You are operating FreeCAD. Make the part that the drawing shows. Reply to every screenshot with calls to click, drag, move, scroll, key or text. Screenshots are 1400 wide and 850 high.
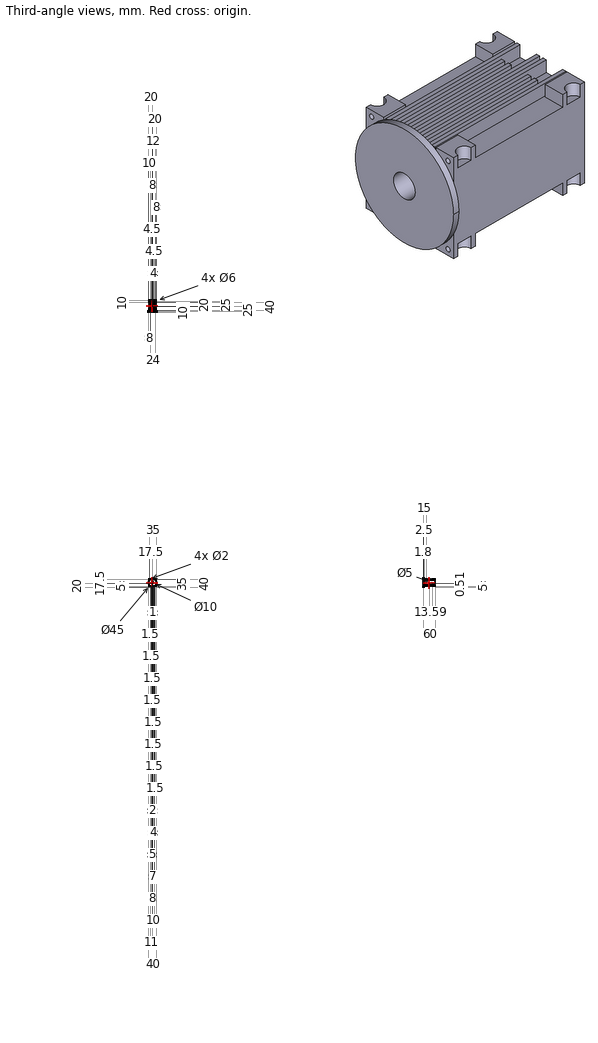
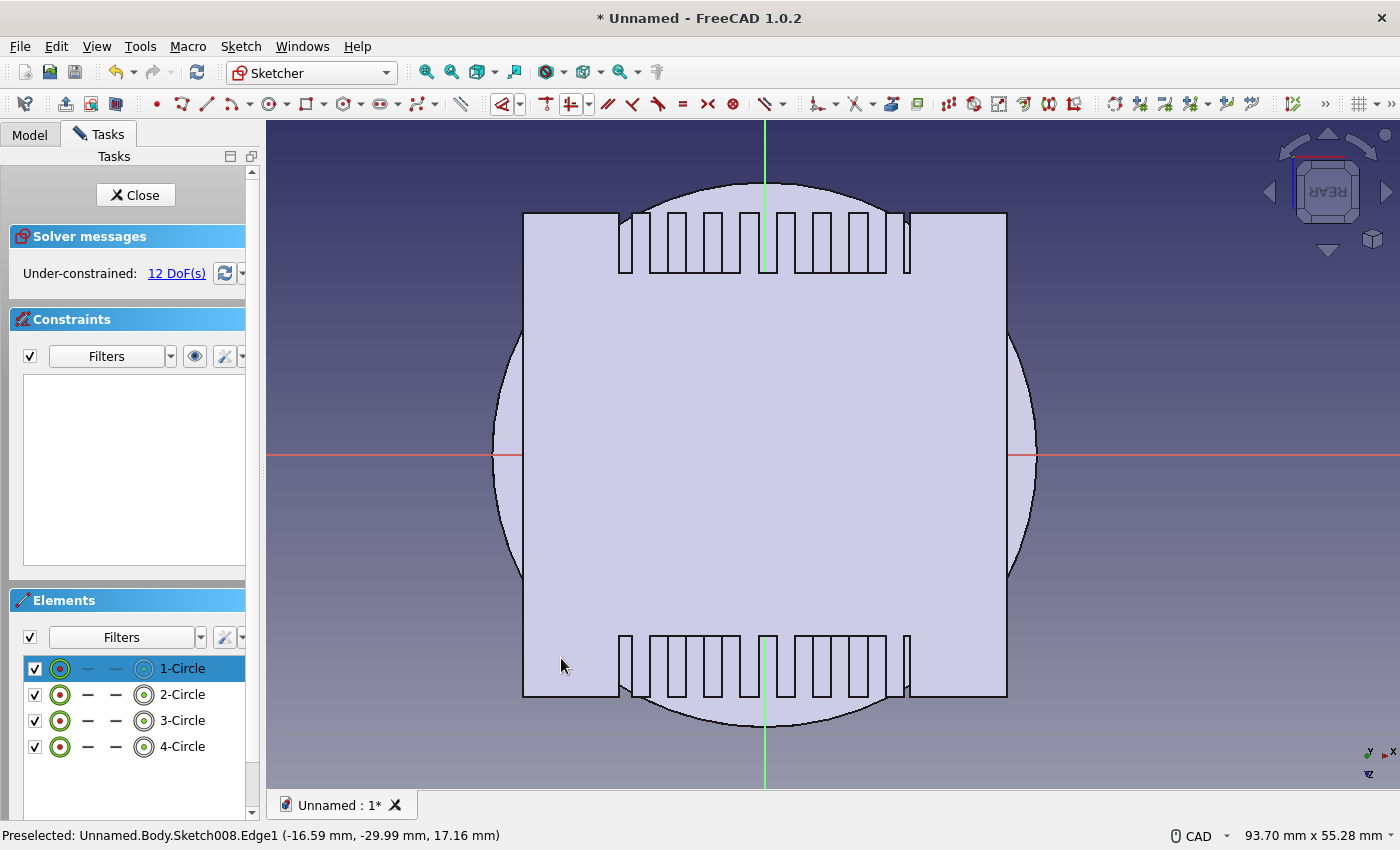
click(985, 658)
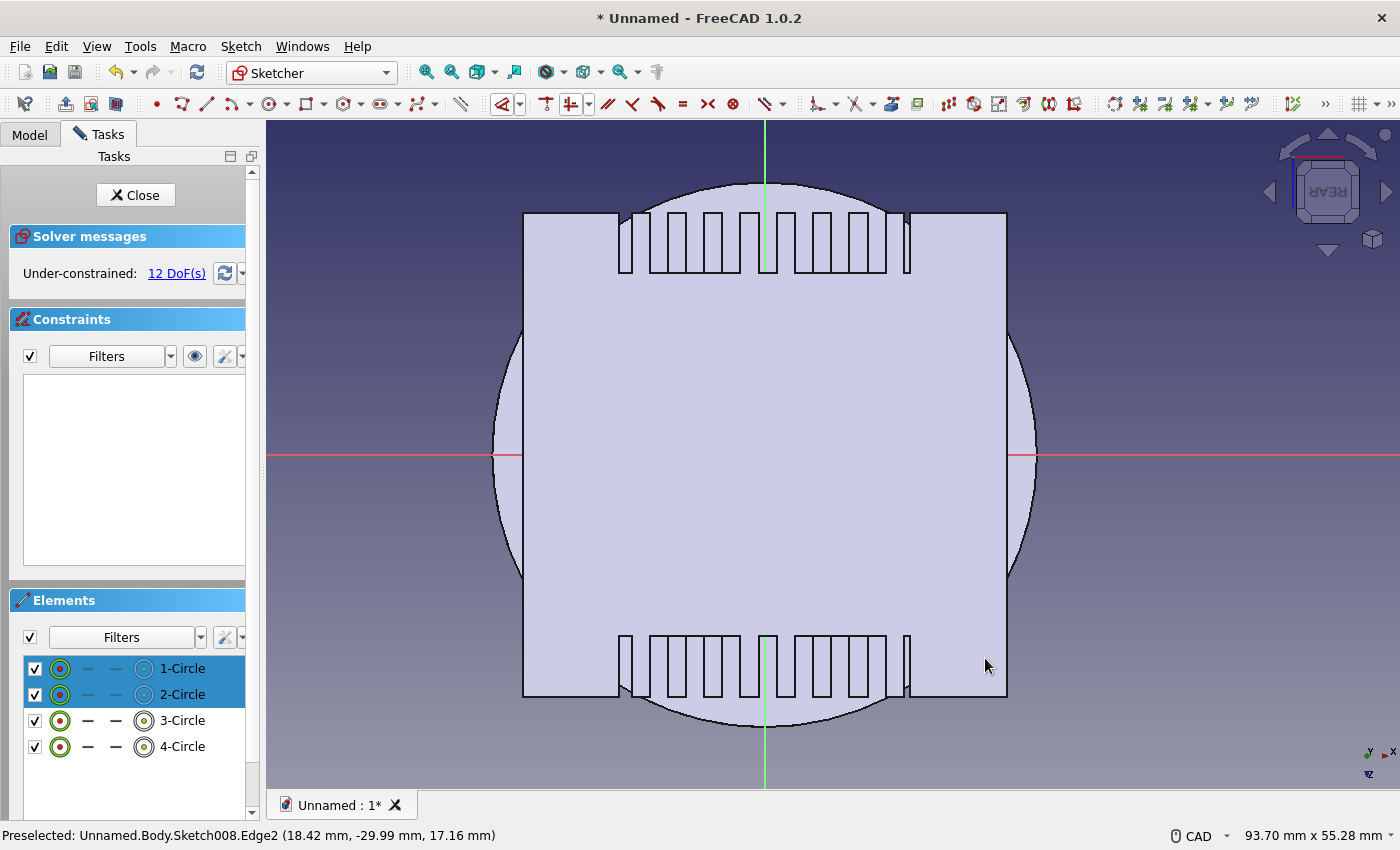
click(985, 235)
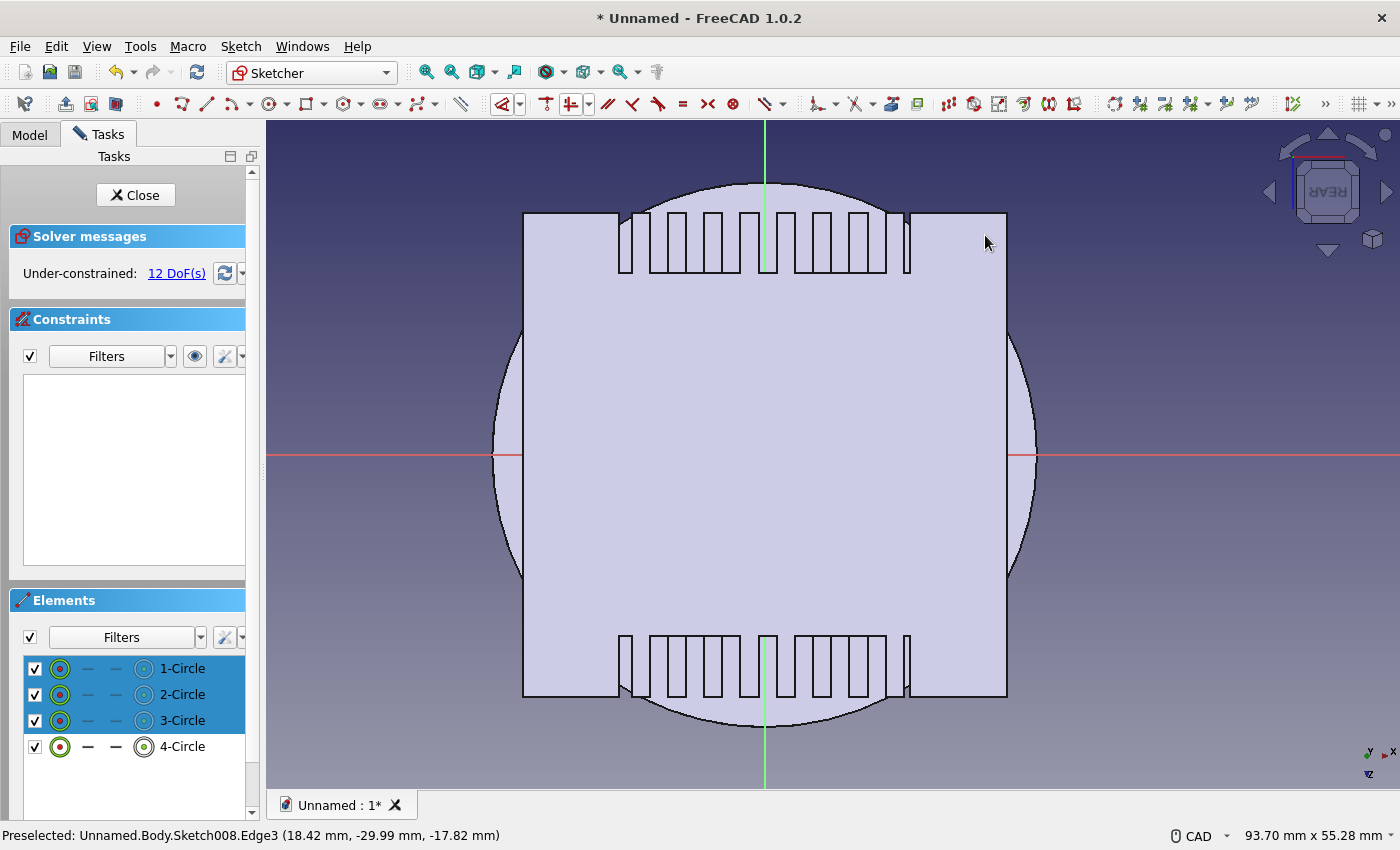
click(561, 235)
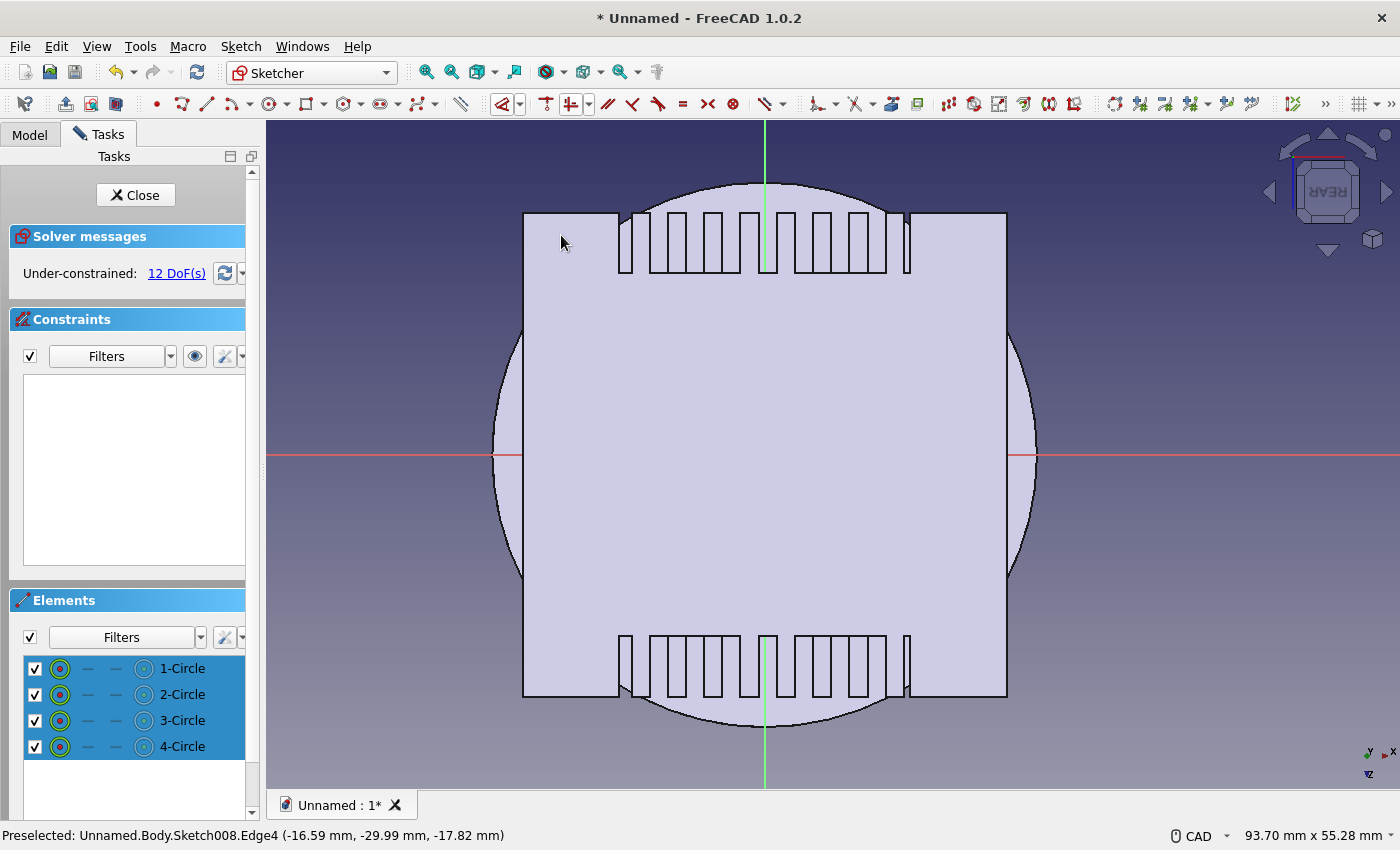
click(683, 104)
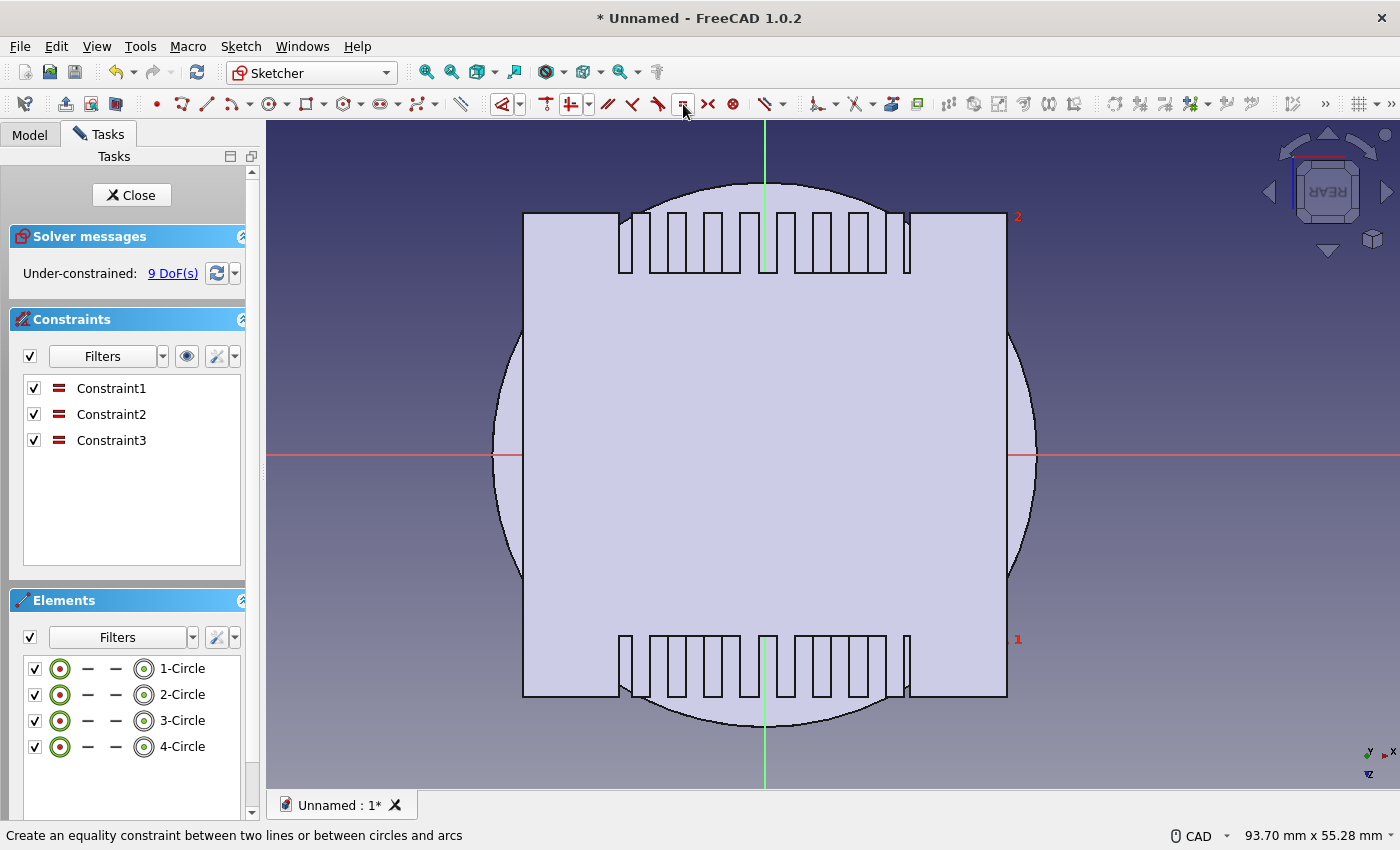
click(553, 667)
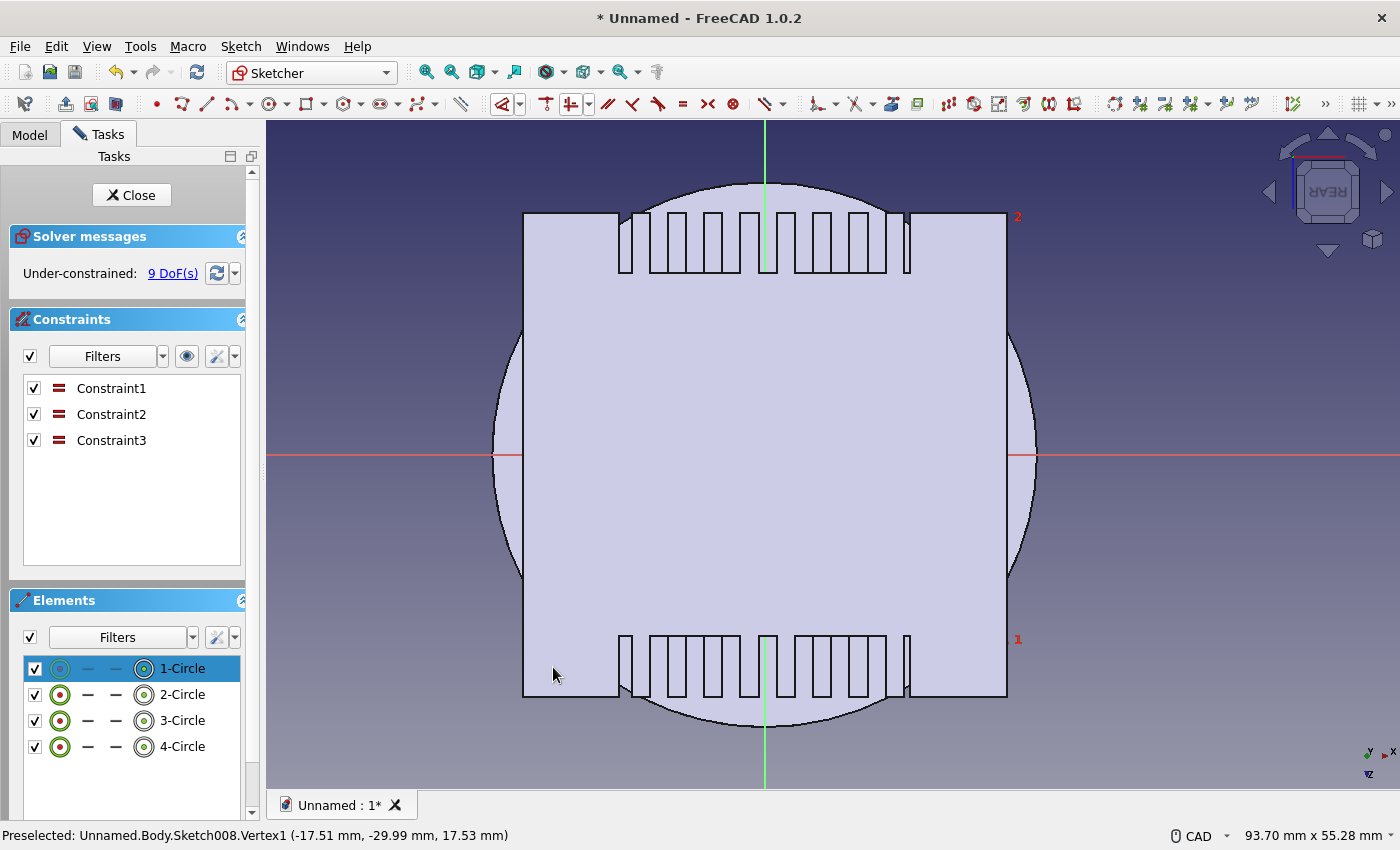
click(976, 667)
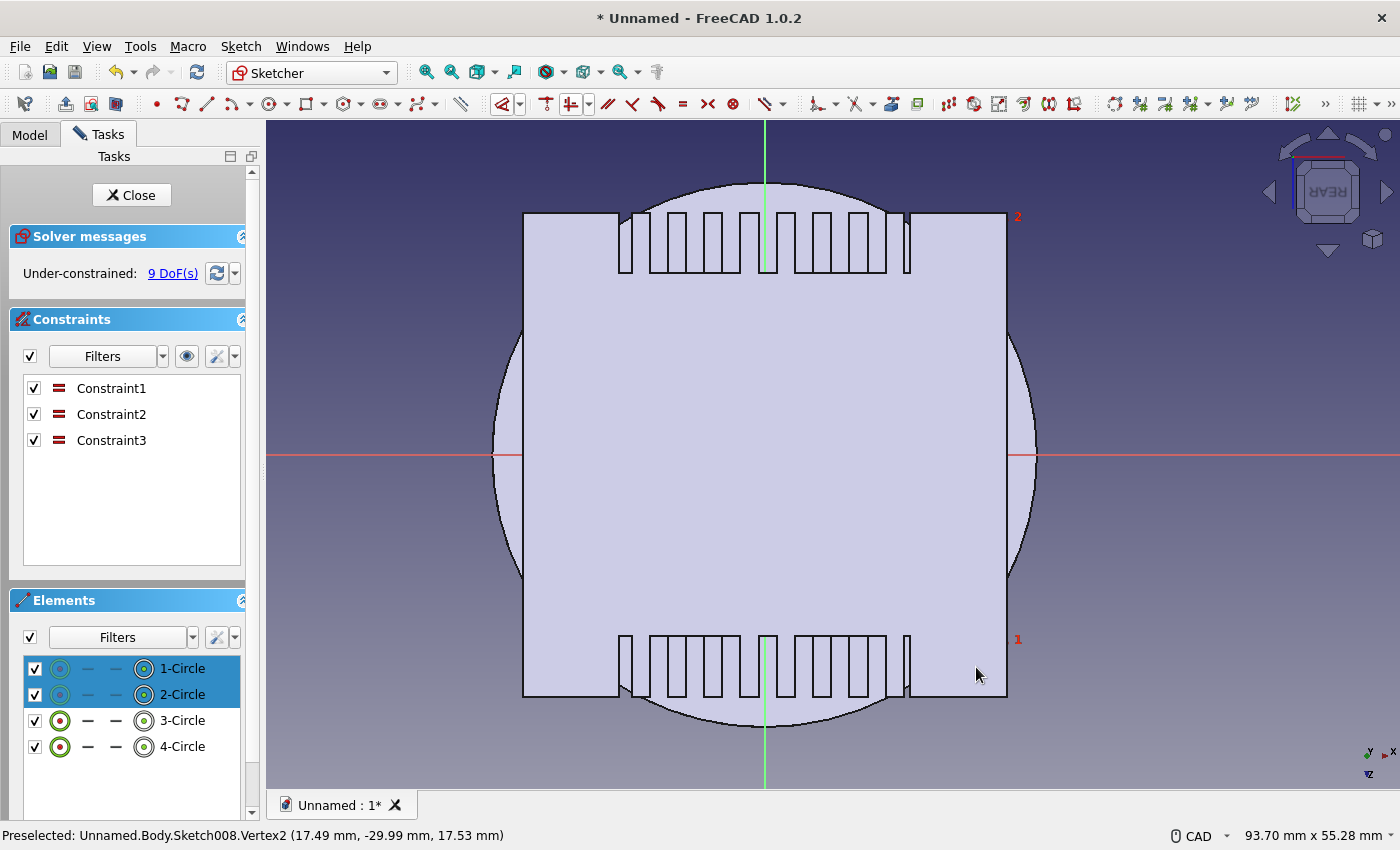
key(h)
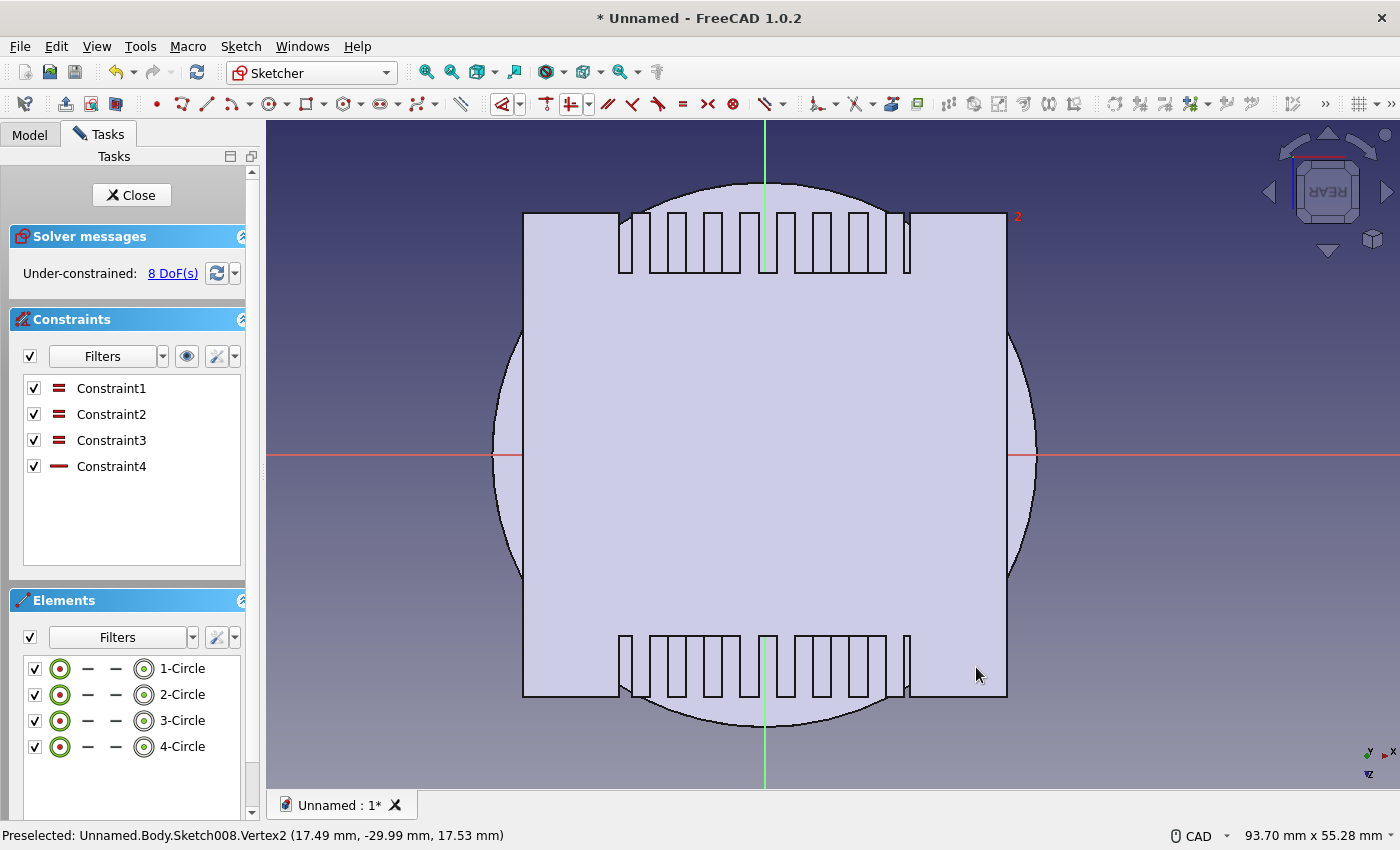
click(976, 667)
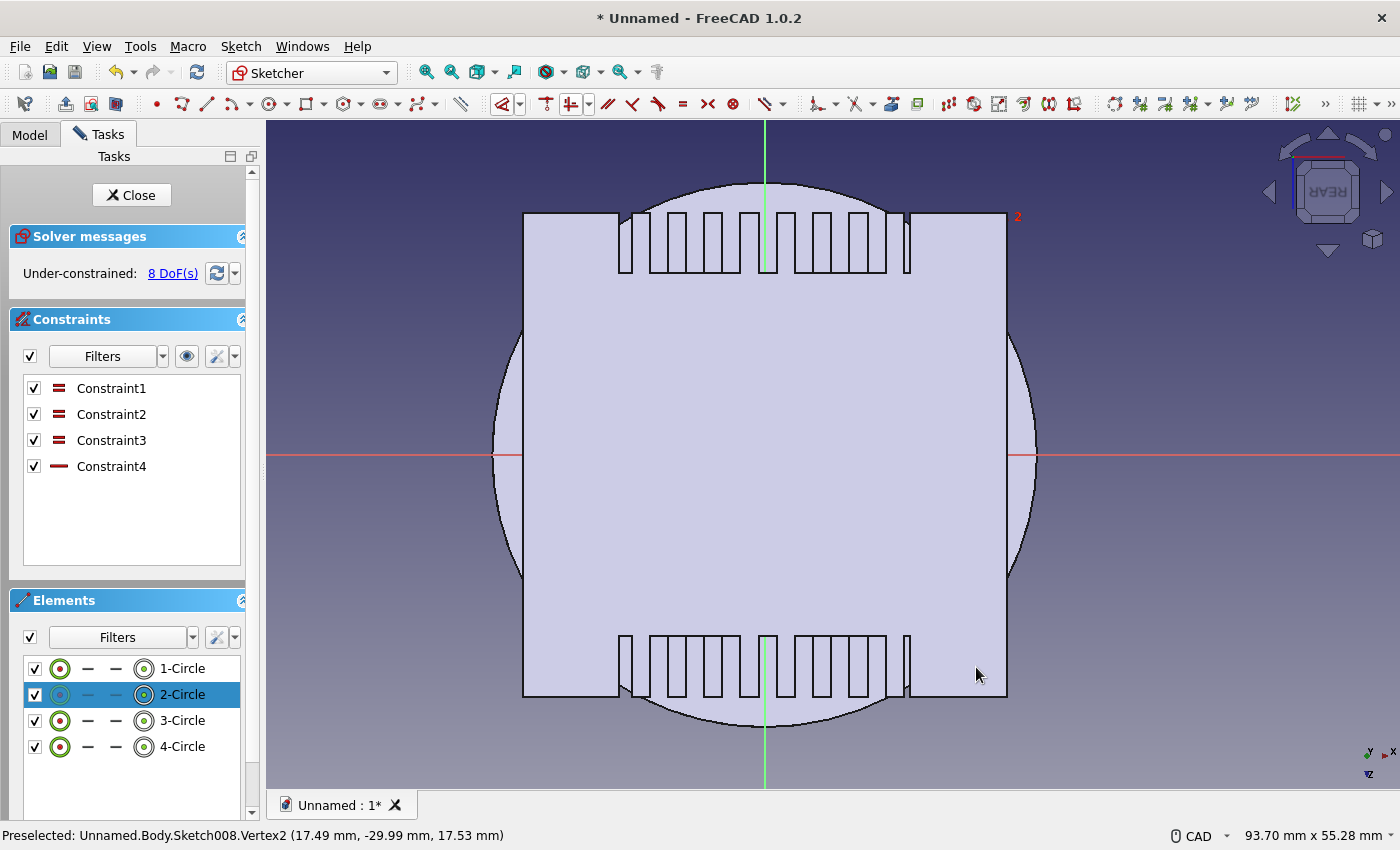
click(976, 244)